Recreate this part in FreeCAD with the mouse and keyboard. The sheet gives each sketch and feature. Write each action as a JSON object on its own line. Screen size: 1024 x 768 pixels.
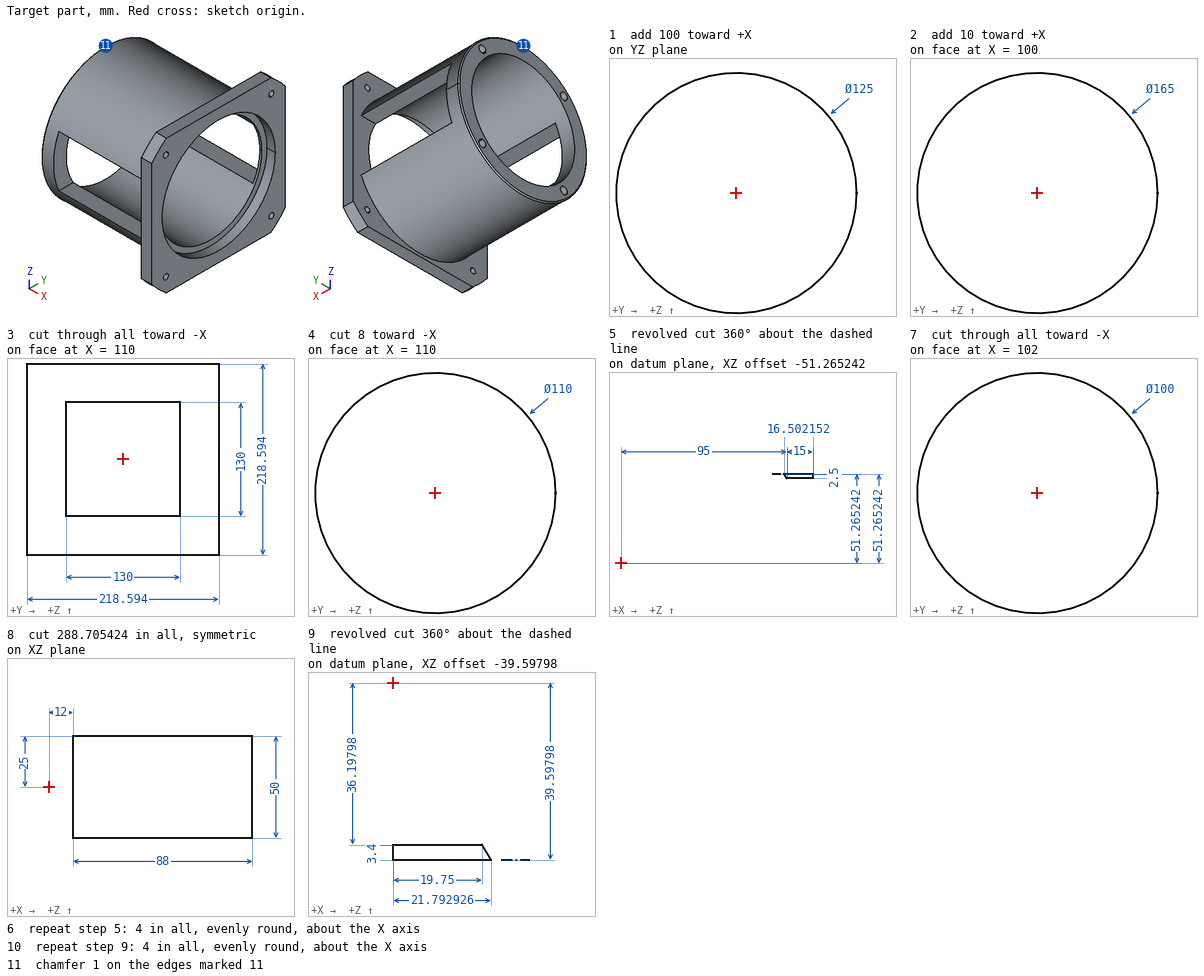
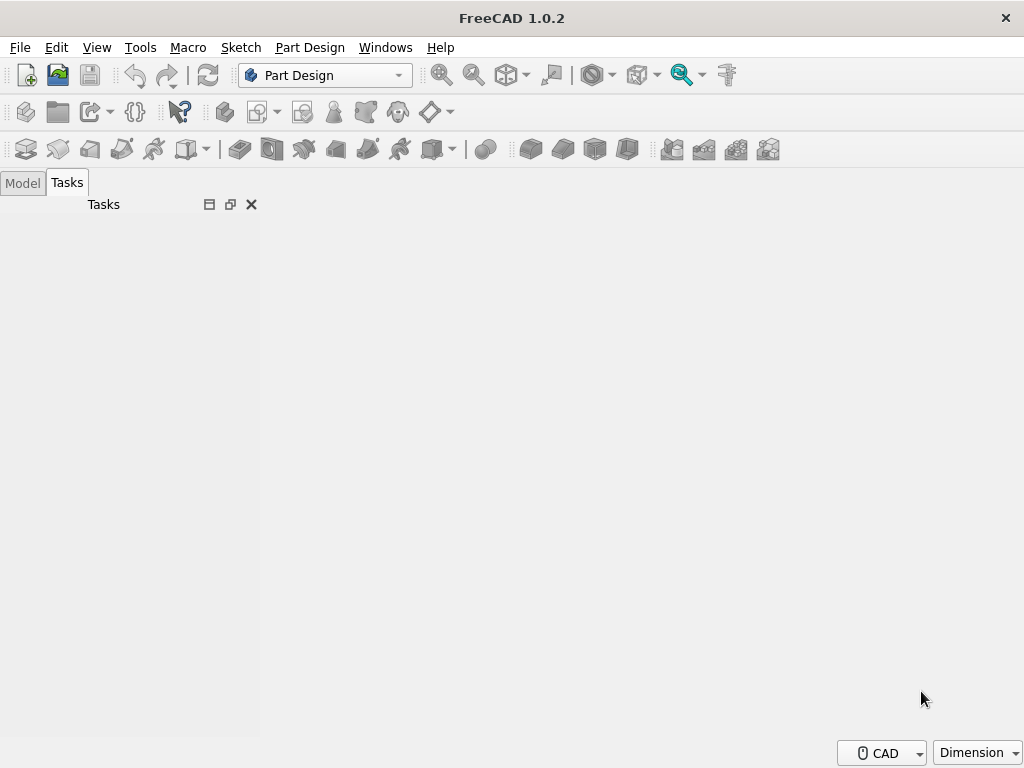
{"action": "left_click", "coordinate": [26, 76]}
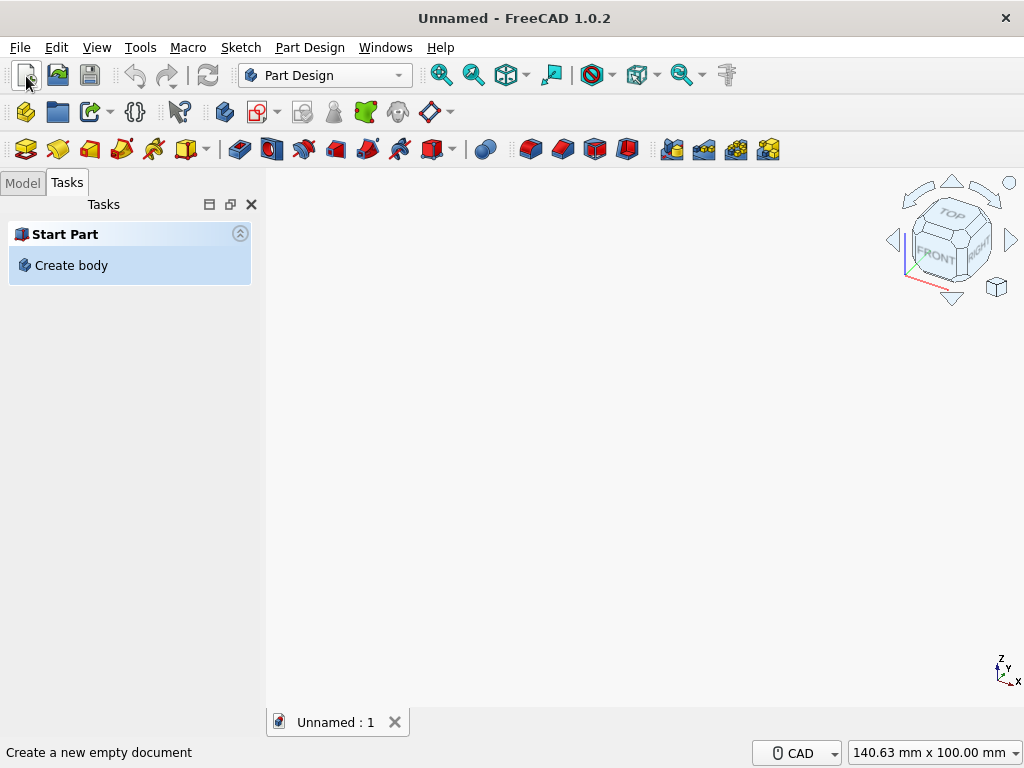
{"action": "left_click", "coordinate": [258, 112]}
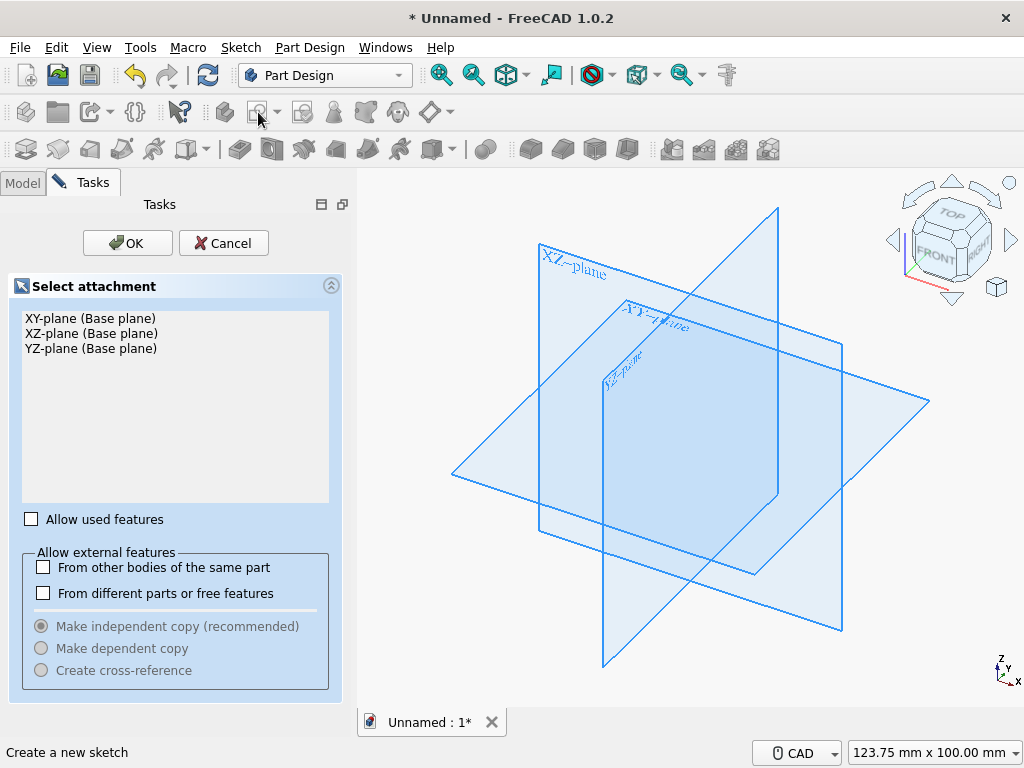
{"action": "left_click", "coordinate": [82, 348]}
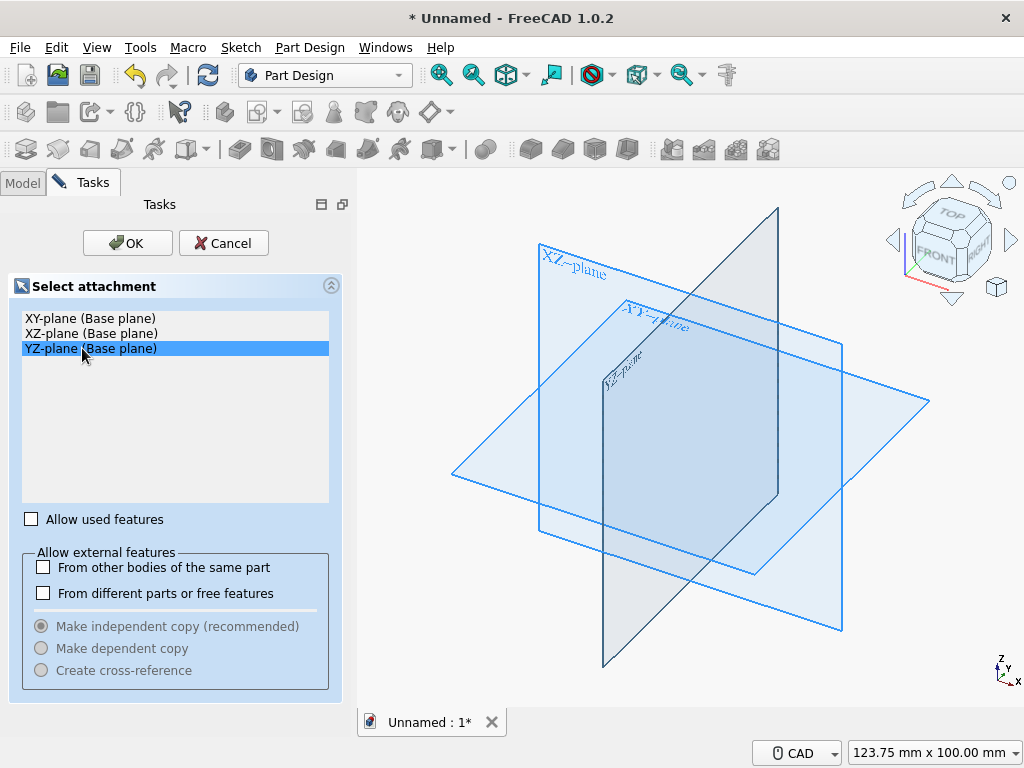
{"action": "left_click", "coordinate": [128, 243]}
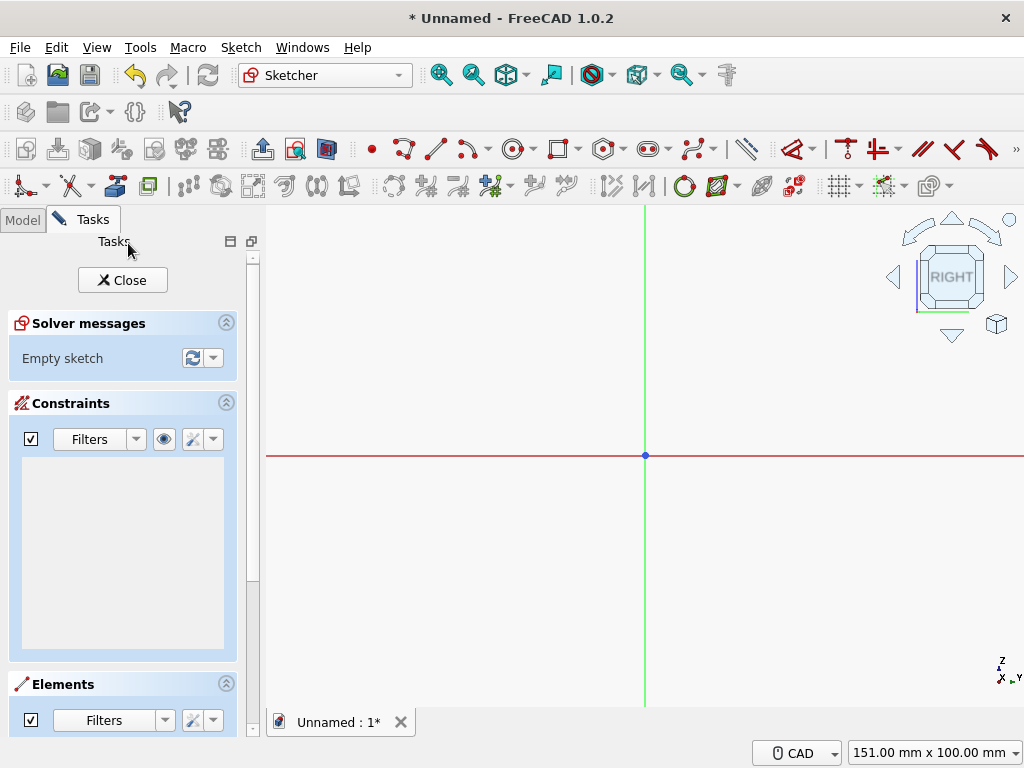
{"action": "scroll", "coordinate": [493, 456], "scroll_direction": "down", "scroll_amount": 3}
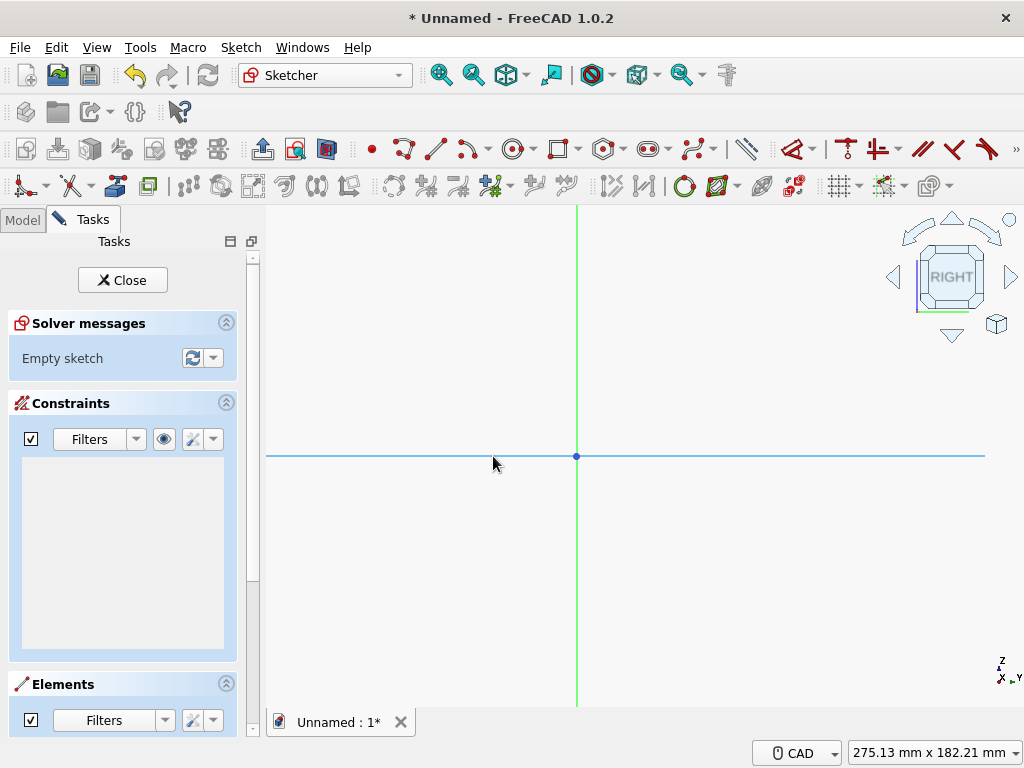
{"action": "left_click", "coordinate": [514, 150]}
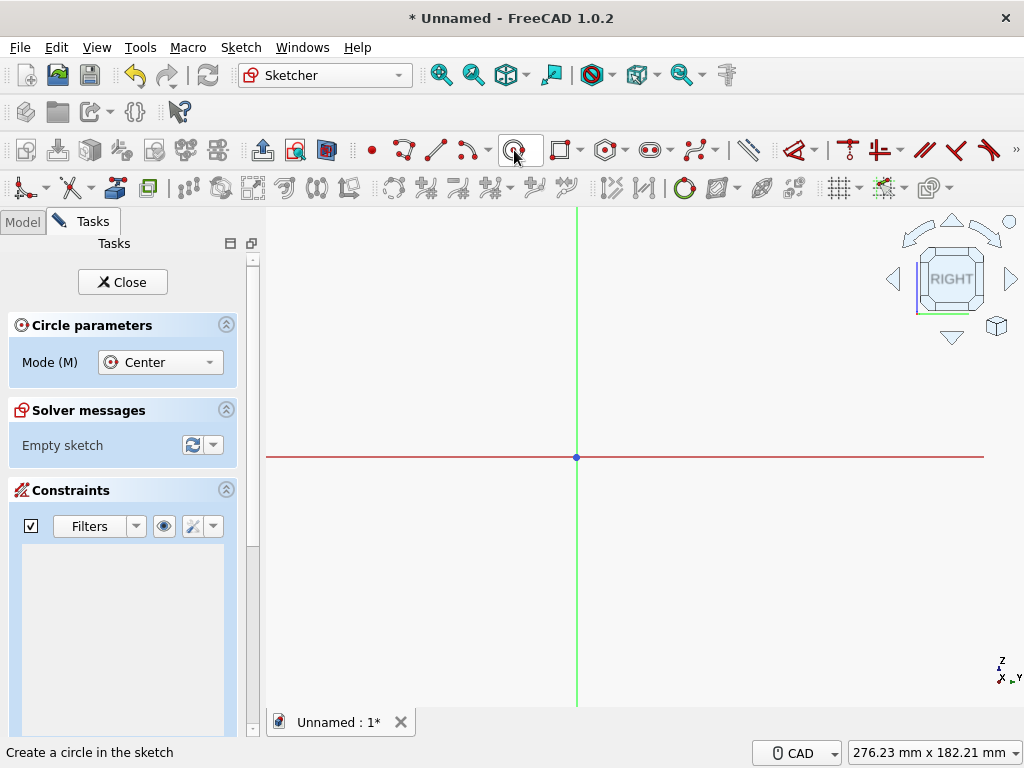
{"action": "left_click", "coordinate": [577, 457]}
{"action": "mouse_move", "coordinate": [698, 336]}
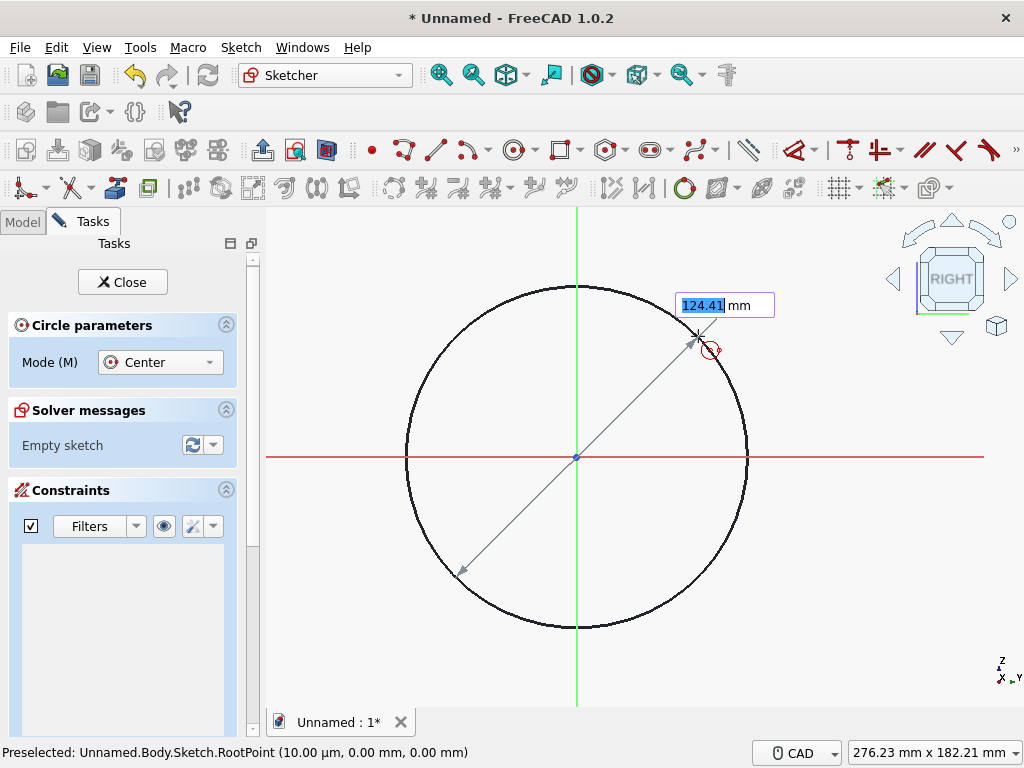
{"action": "type", "text": "125"}
{"action": "key", "text": "Return"}
{"action": "key", "text": "Escape"}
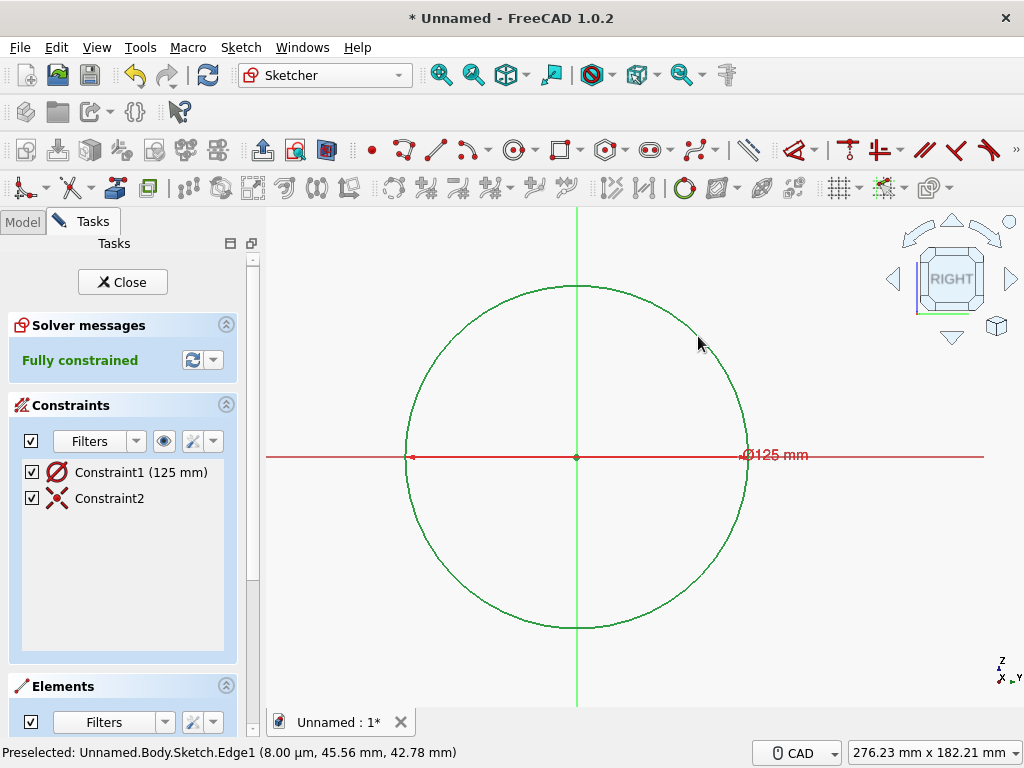
{"action": "left_click", "coordinate": [123, 282]}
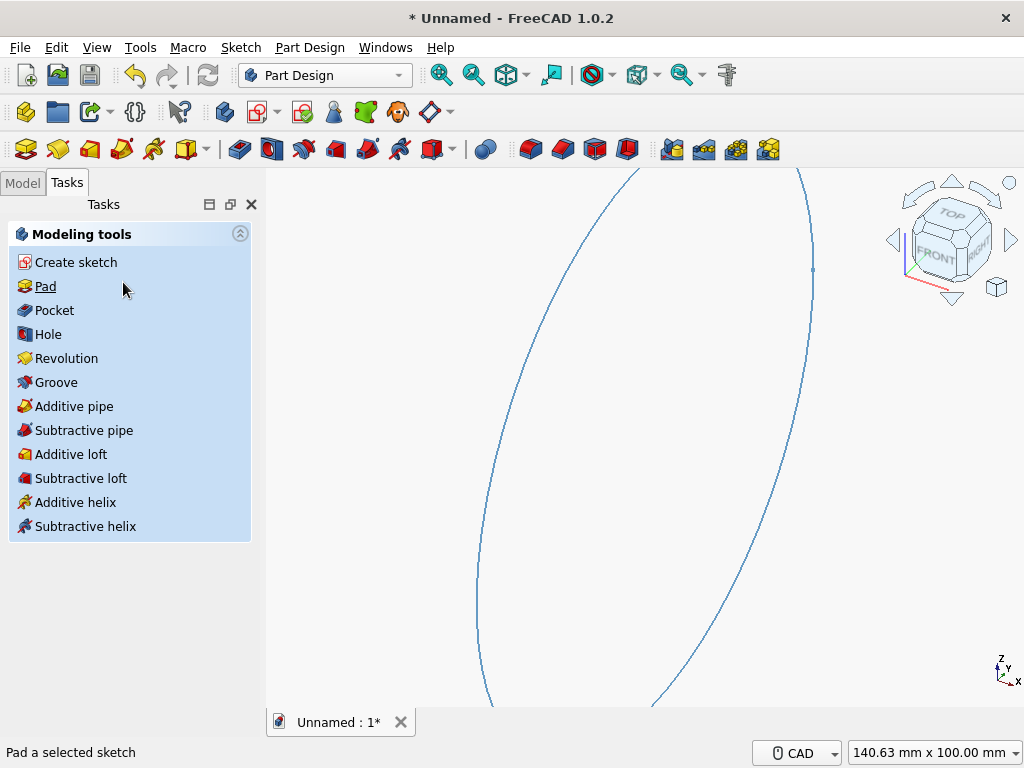
{"action": "left_click", "coordinate": [26, 150]}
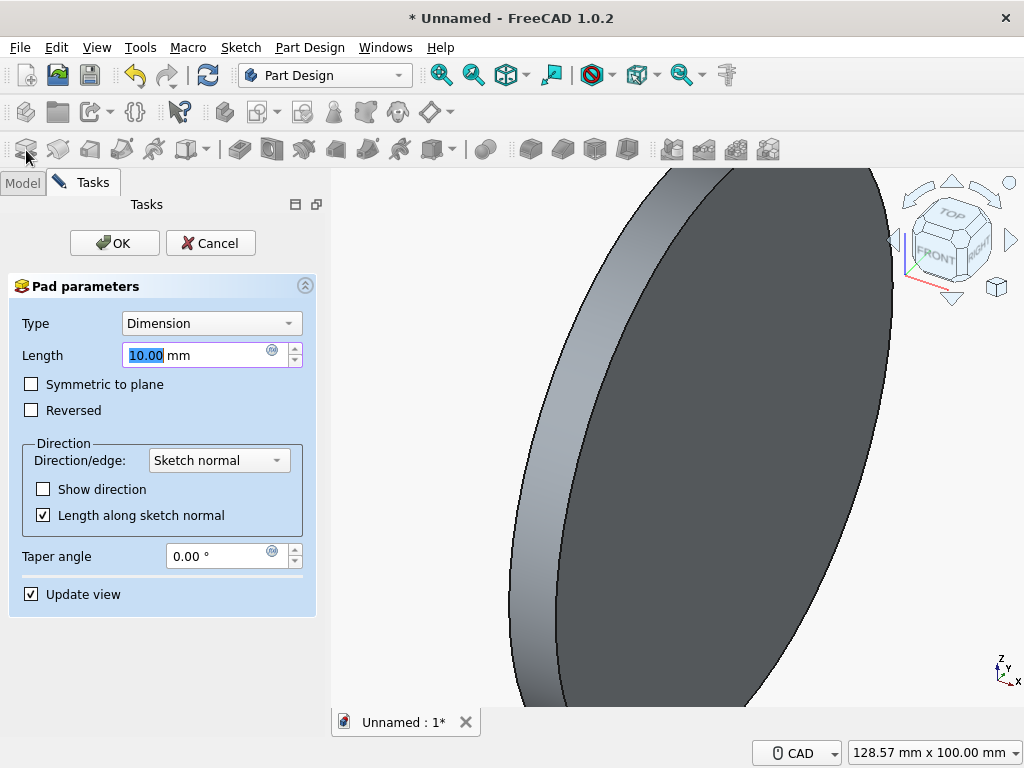
{"action": "type", "text": "100"}
{"action": "key", "text": "Tab"}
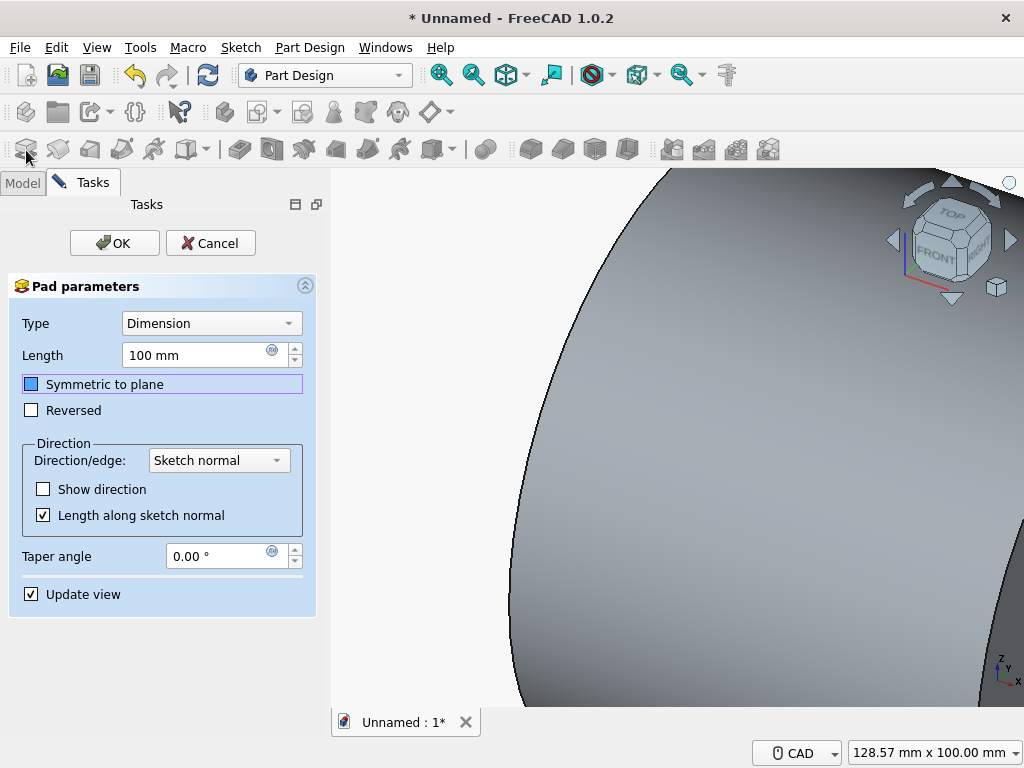
{"action": "left_click", "coordinate": [115, 243]}